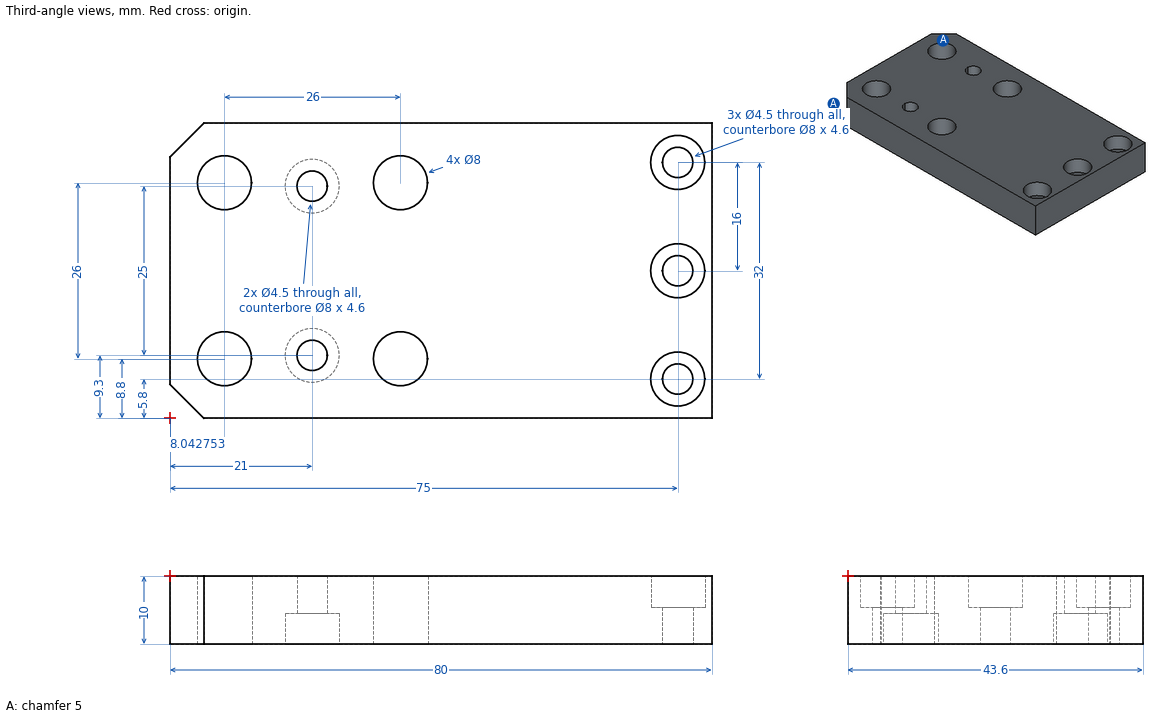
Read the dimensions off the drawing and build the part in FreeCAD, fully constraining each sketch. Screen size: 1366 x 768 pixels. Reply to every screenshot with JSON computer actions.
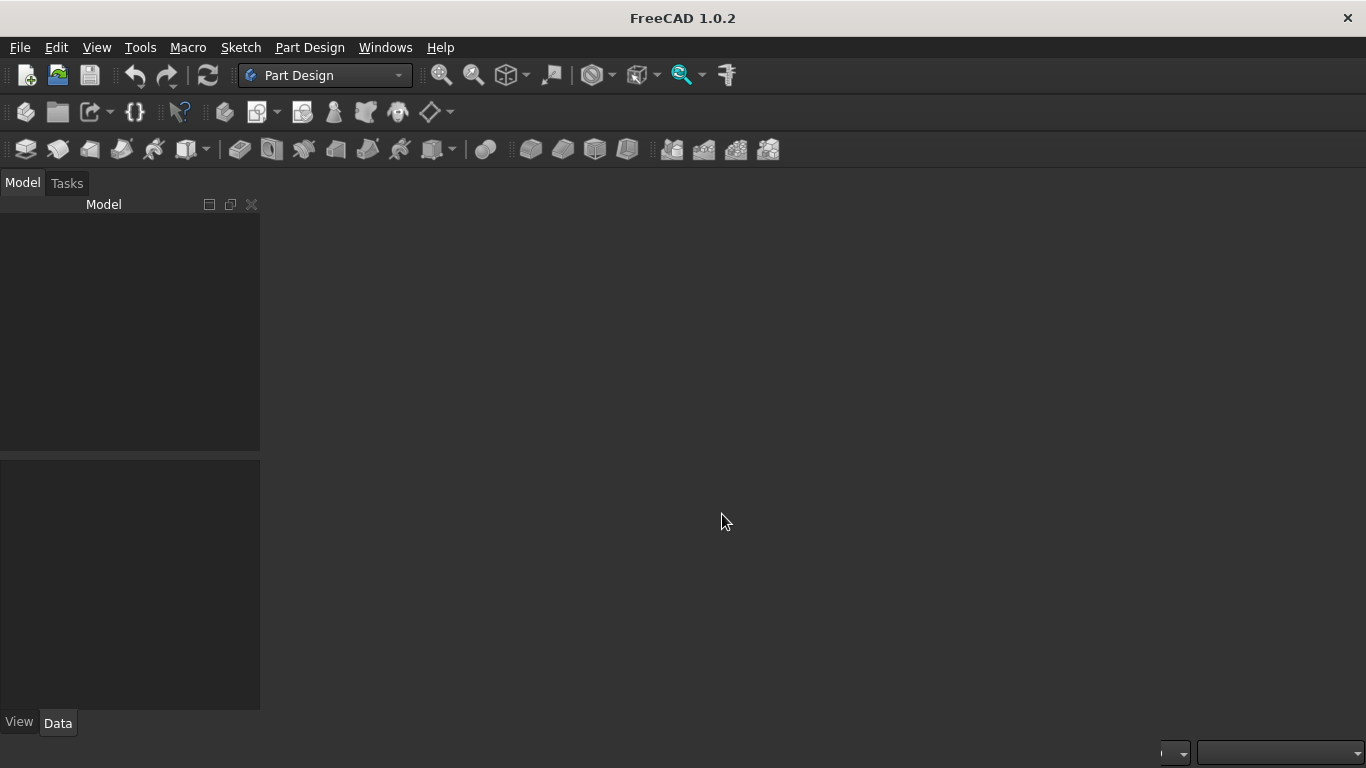
{"action": "left_click", "coordinate": [26, 76]}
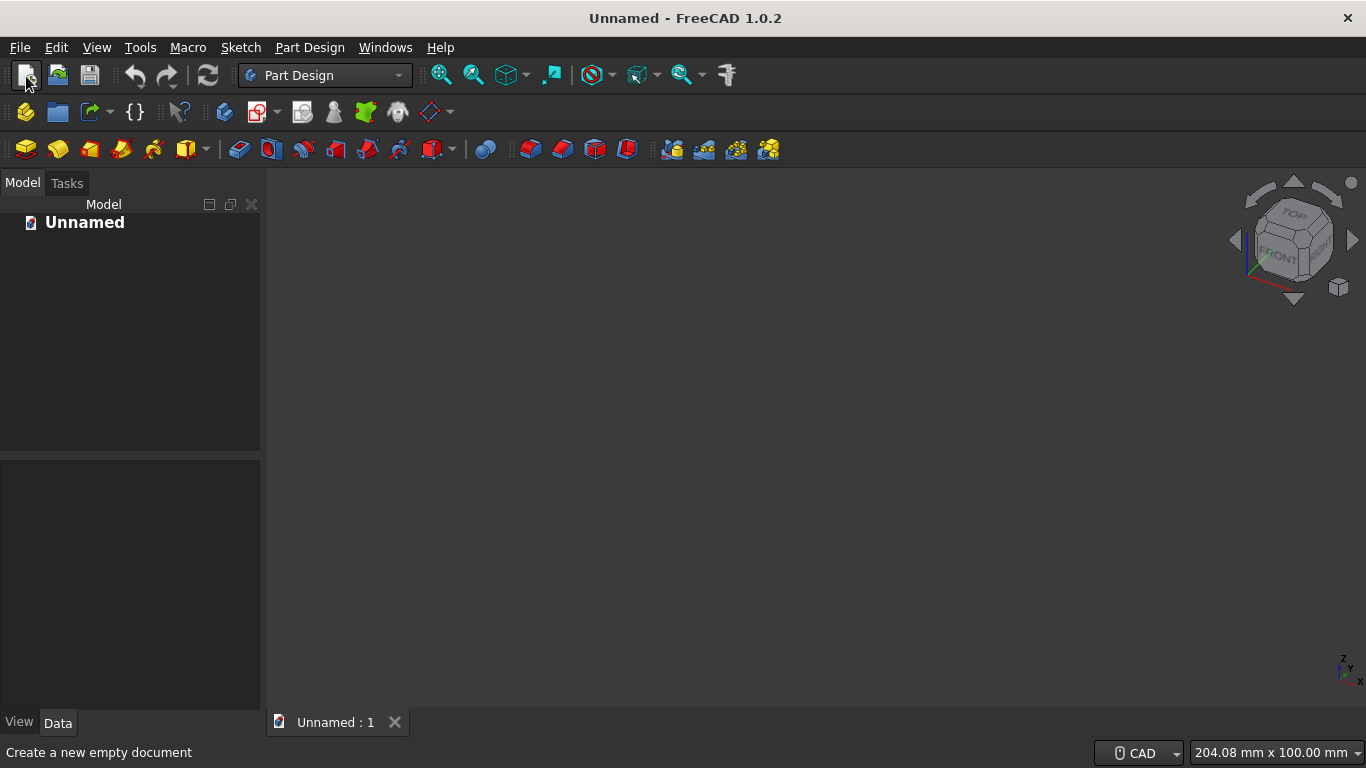
{"action": "left_click", "coordinate": [258, 112]}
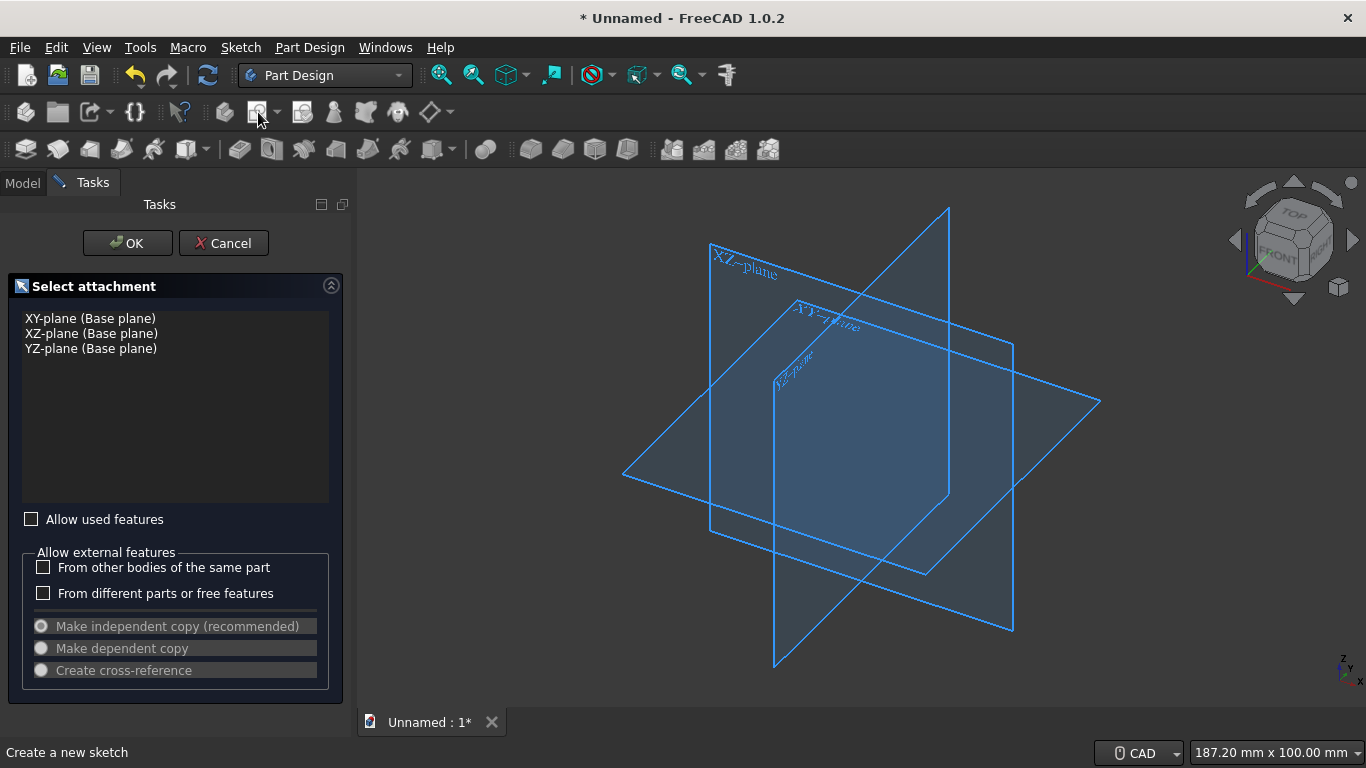
{"action": "left_click", "coordinate": [82, 334]}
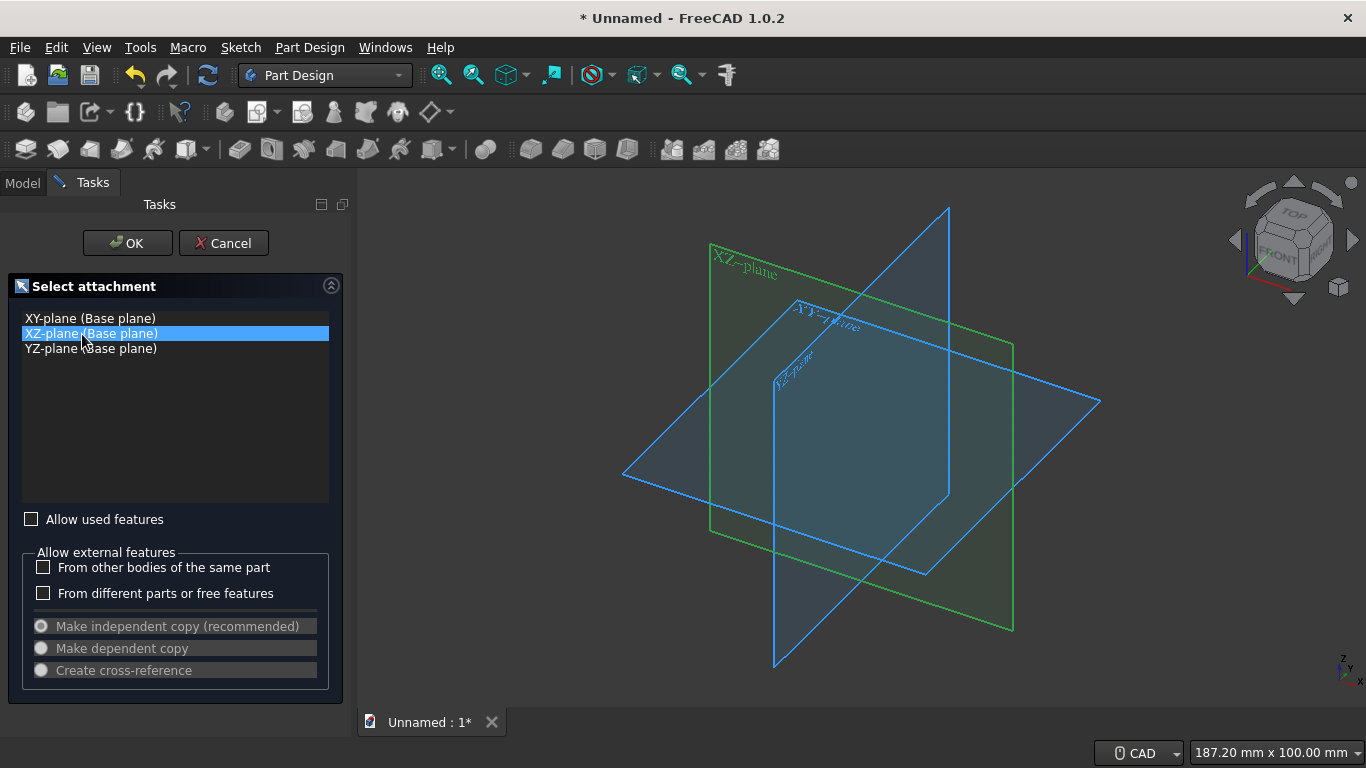
{"action": "left_click", "coordinate": [128, 243]}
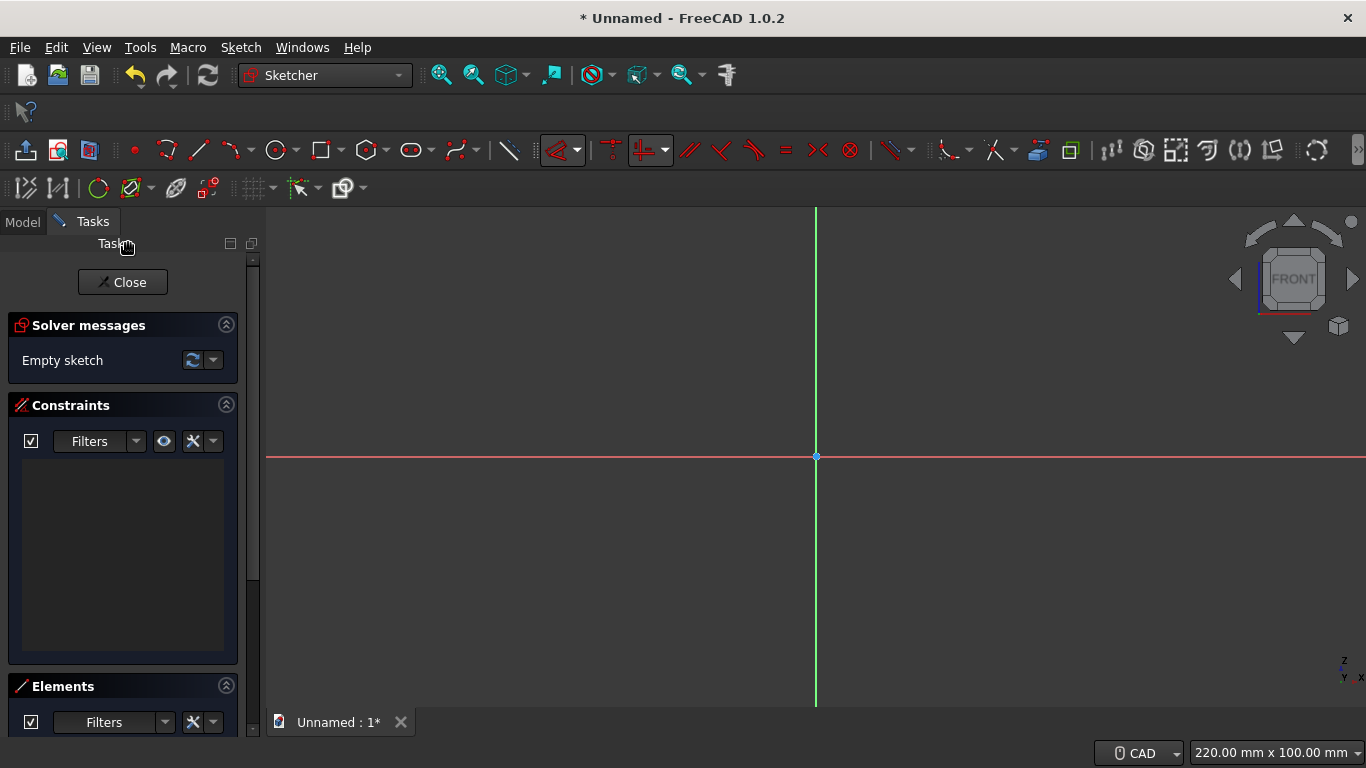
{"action": "scroll", "coordinate": [294, 344], "scroll_direction": "down", "scroll_amount": 1}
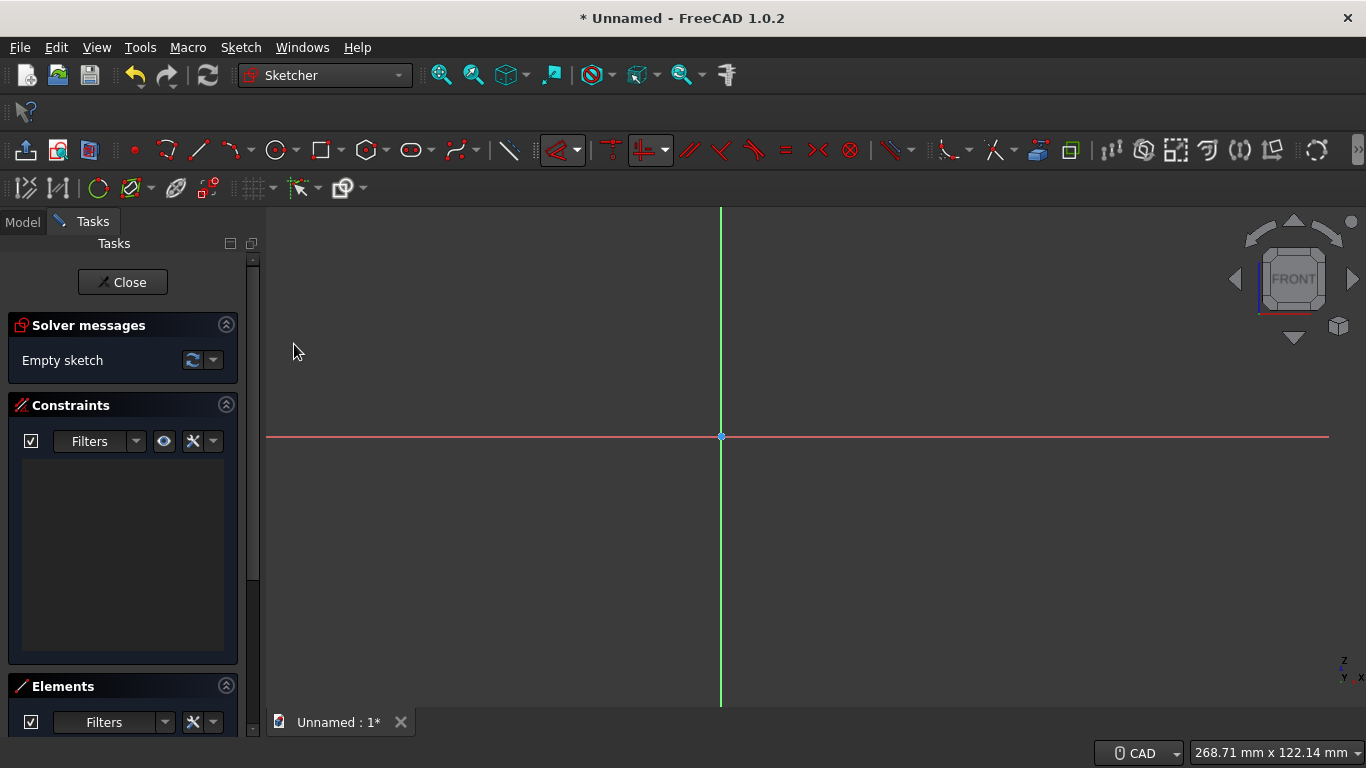
{"action": "scroll", "coordinate": [1053, 457], "scroll_direction": "up", "scroll_amount": 3}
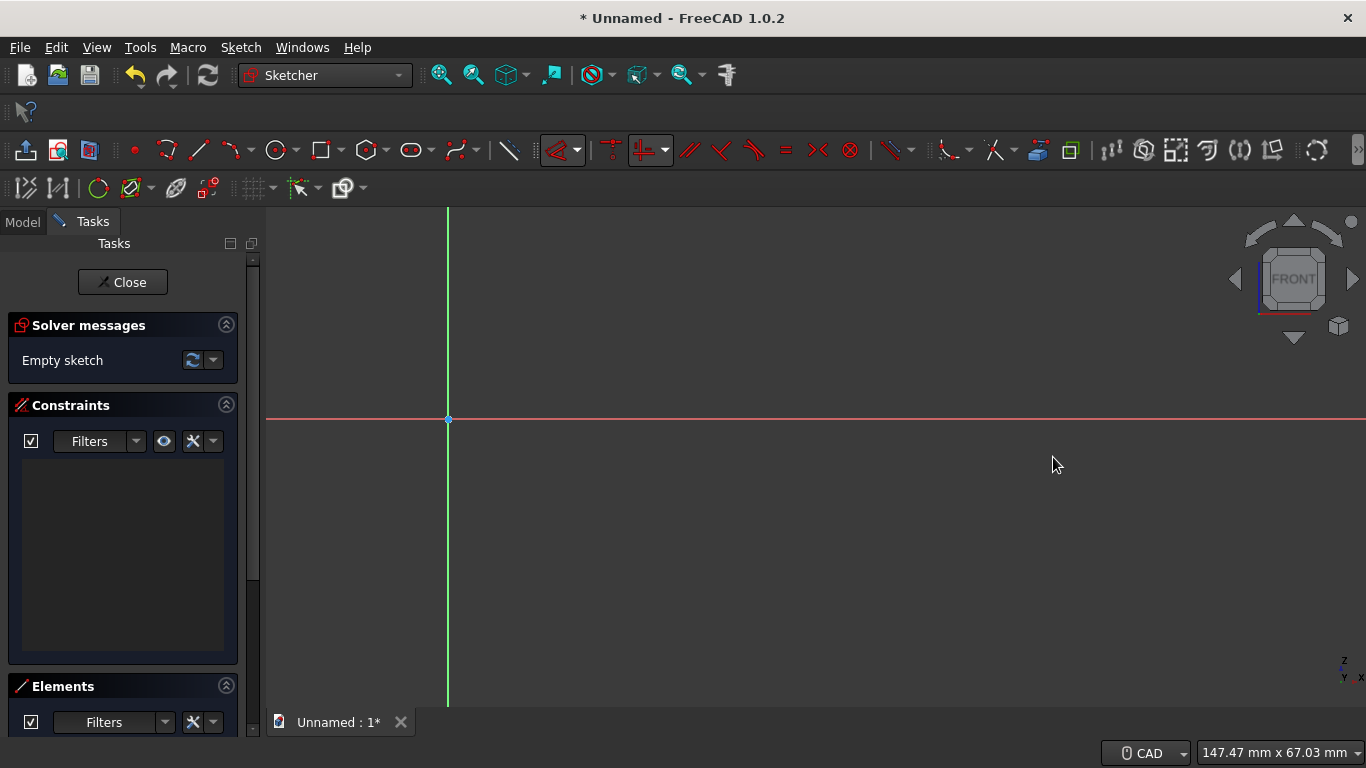
{"action": "left_click", "coordinate": [322, 150]}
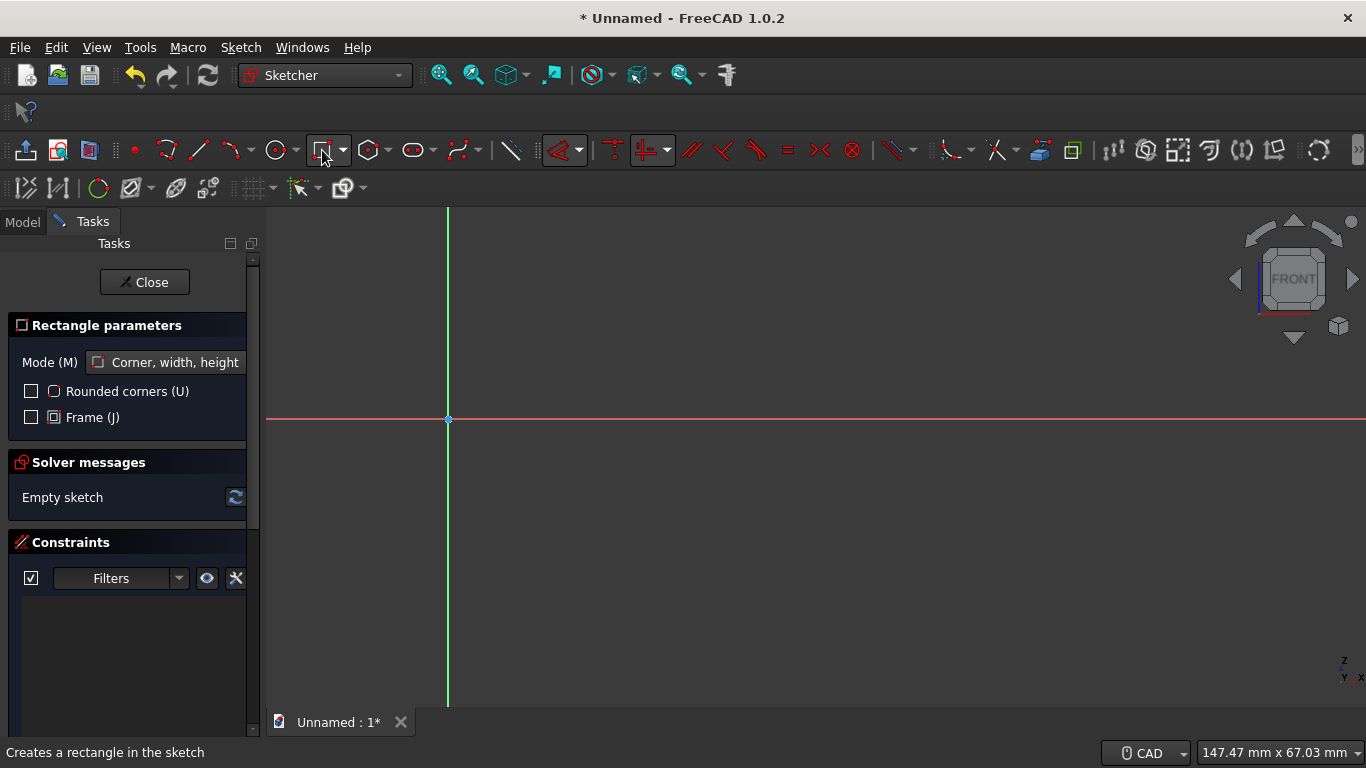
{"action": "left_click", "coordinate": [448, 419]}
{"action": "left_click", "coordinate": [1045, 494]}
{"action": "key", "text": "Escape"}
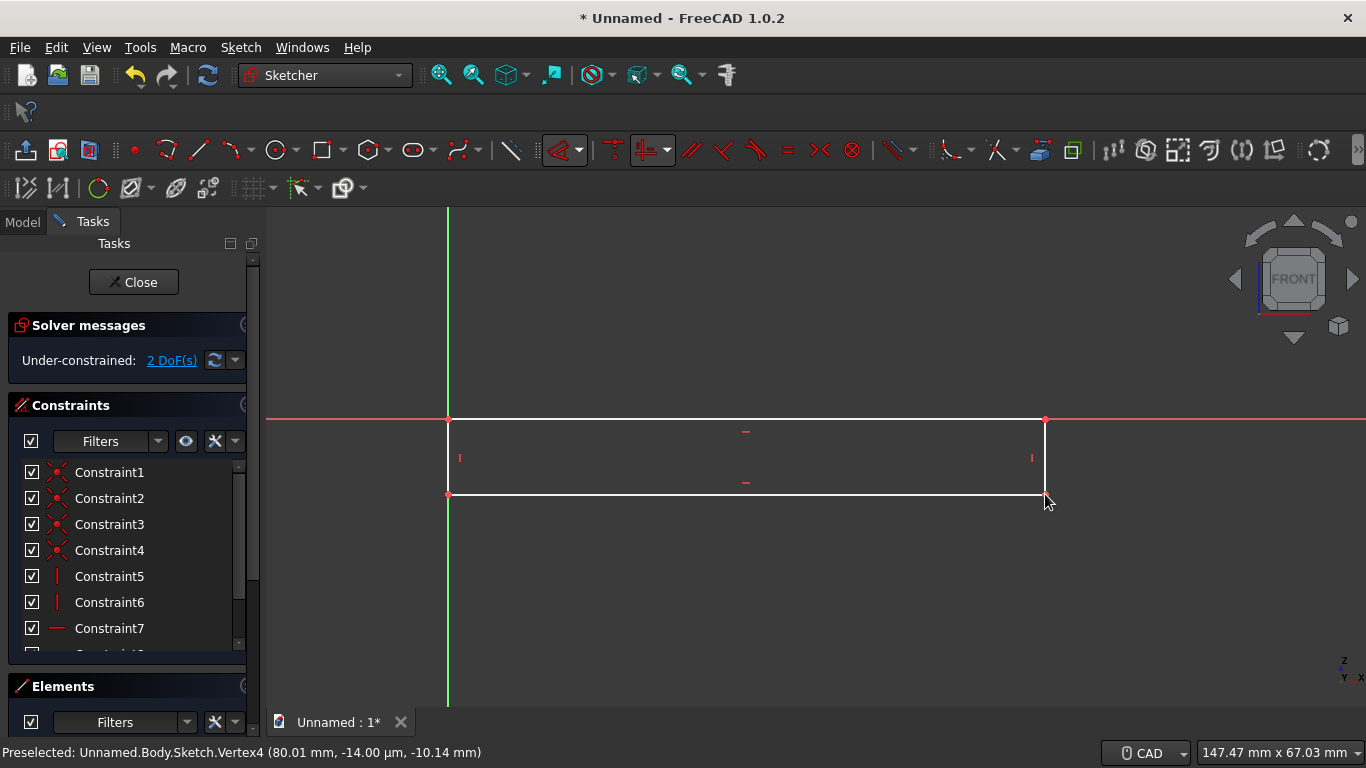
{"action": "left_click", "coordinate": [448, 442]}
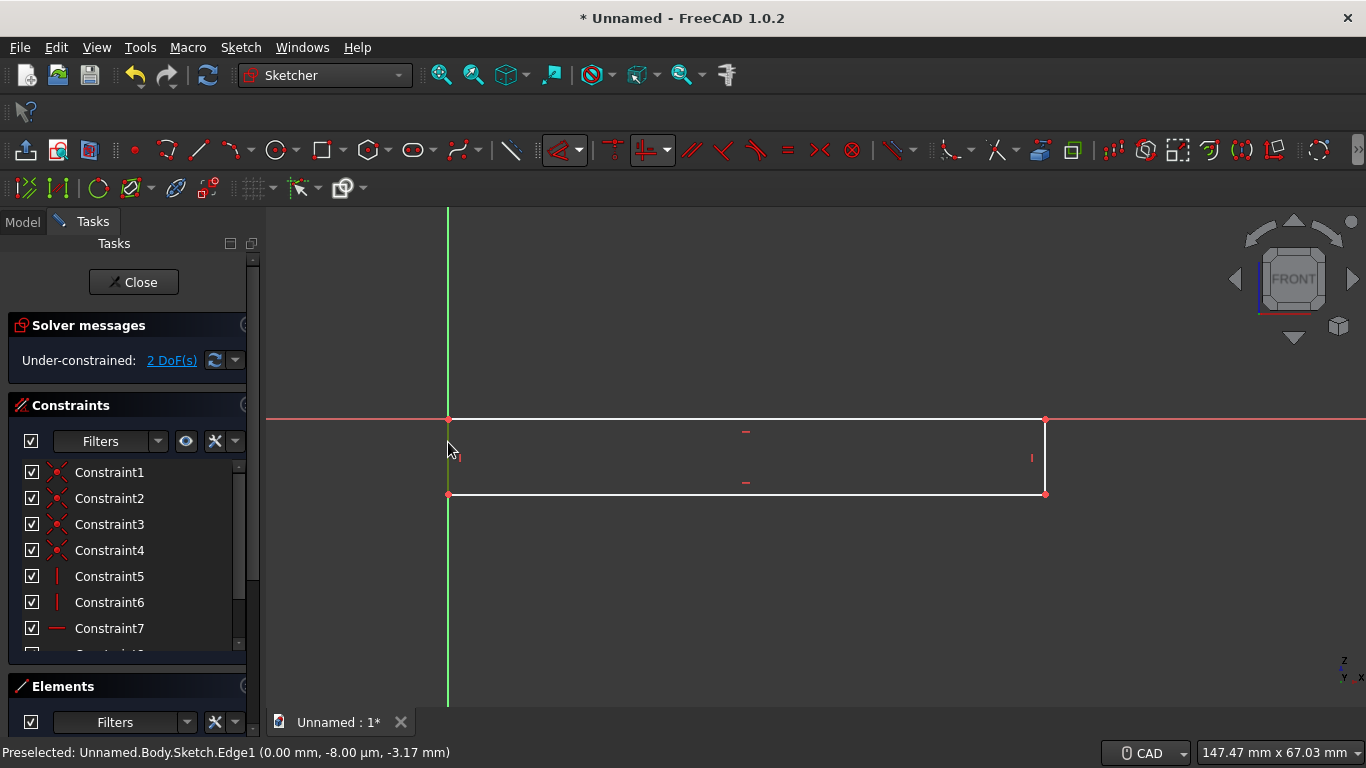
{"action": "left_click", "coordinate": [582, 150]}